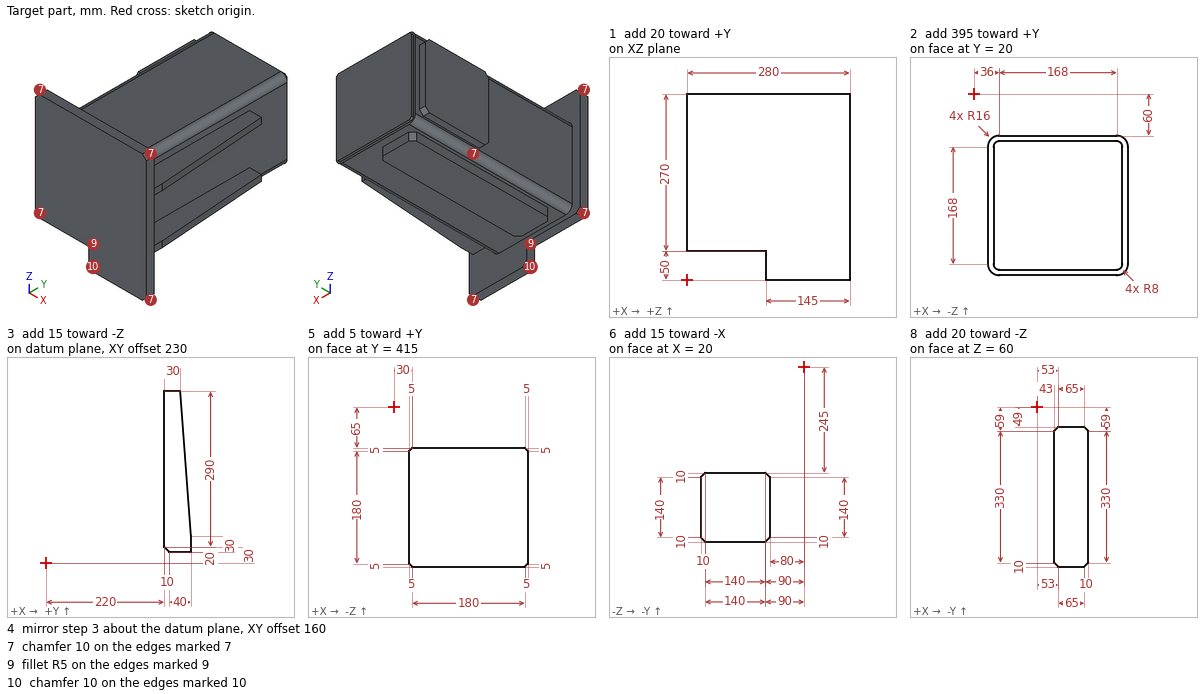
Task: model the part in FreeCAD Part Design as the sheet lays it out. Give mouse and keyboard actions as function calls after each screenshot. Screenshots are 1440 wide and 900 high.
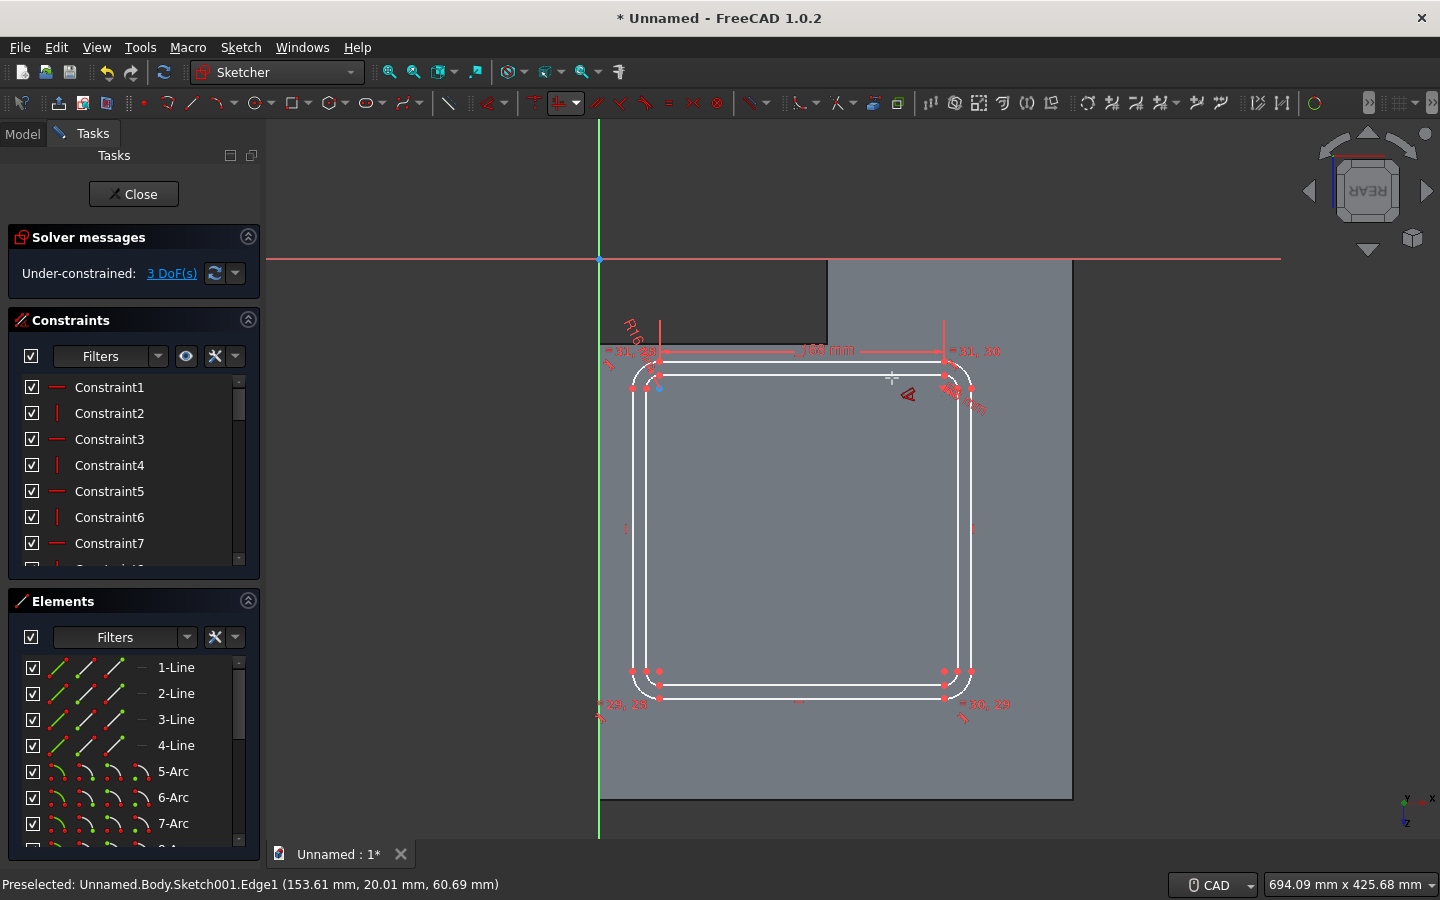
click(633, 474)
click(667, 530)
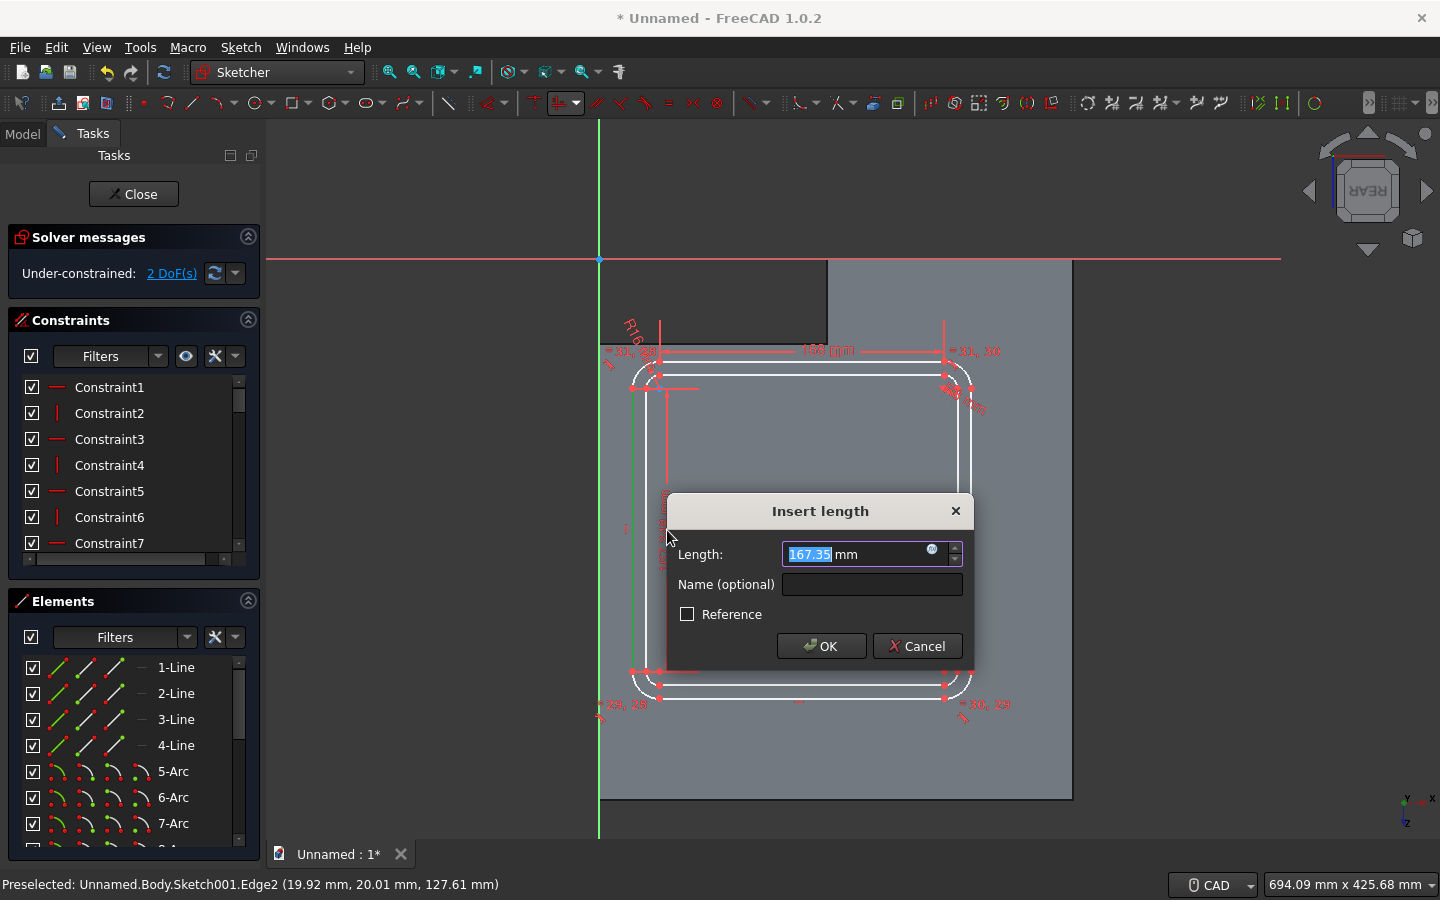
text(168)
key(Return)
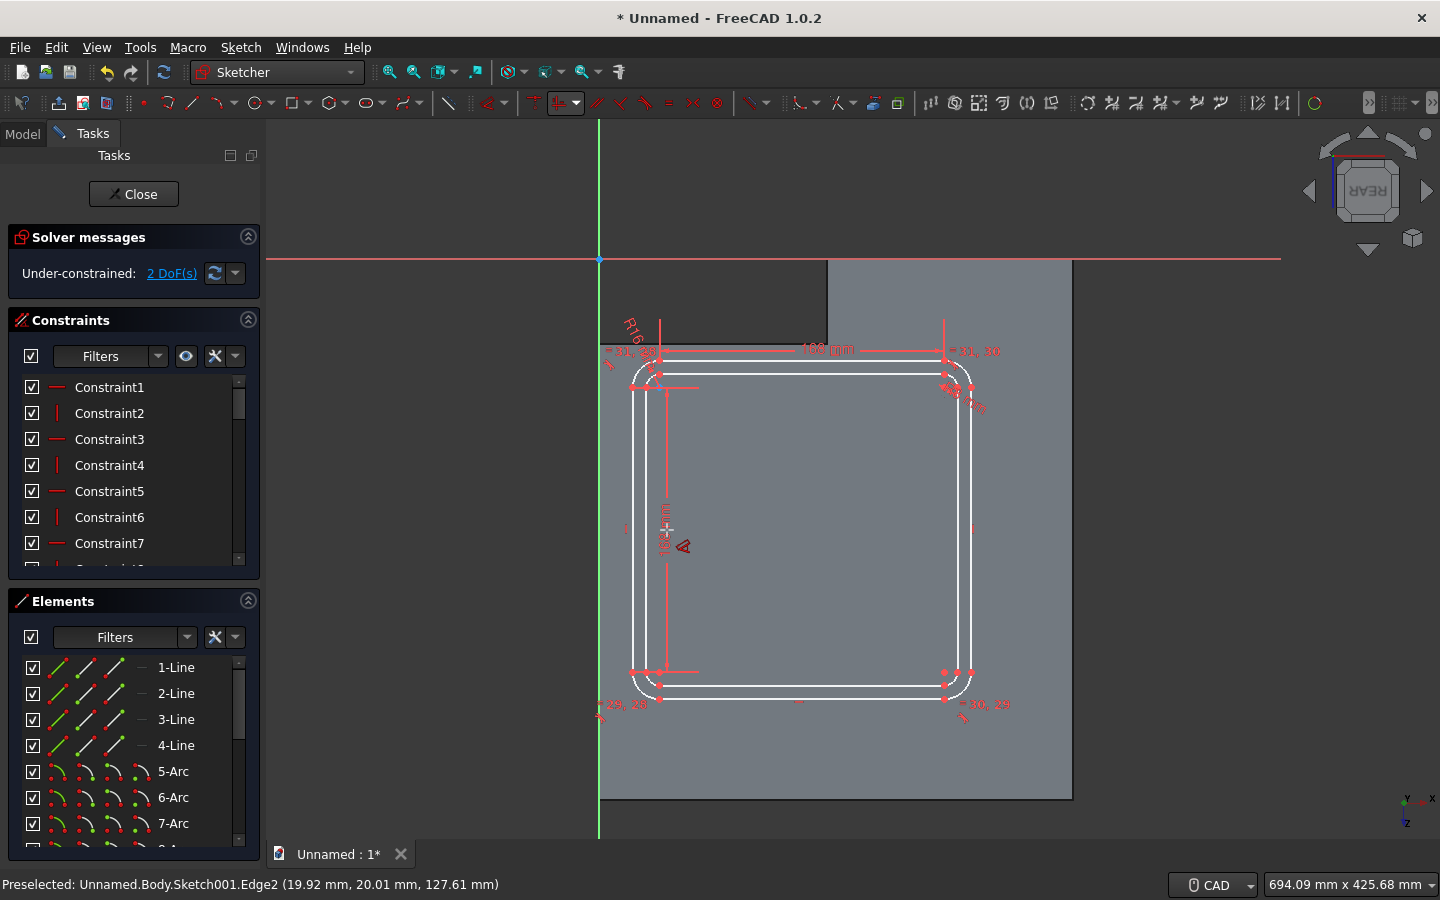
click(944, 361)
click(565, 310)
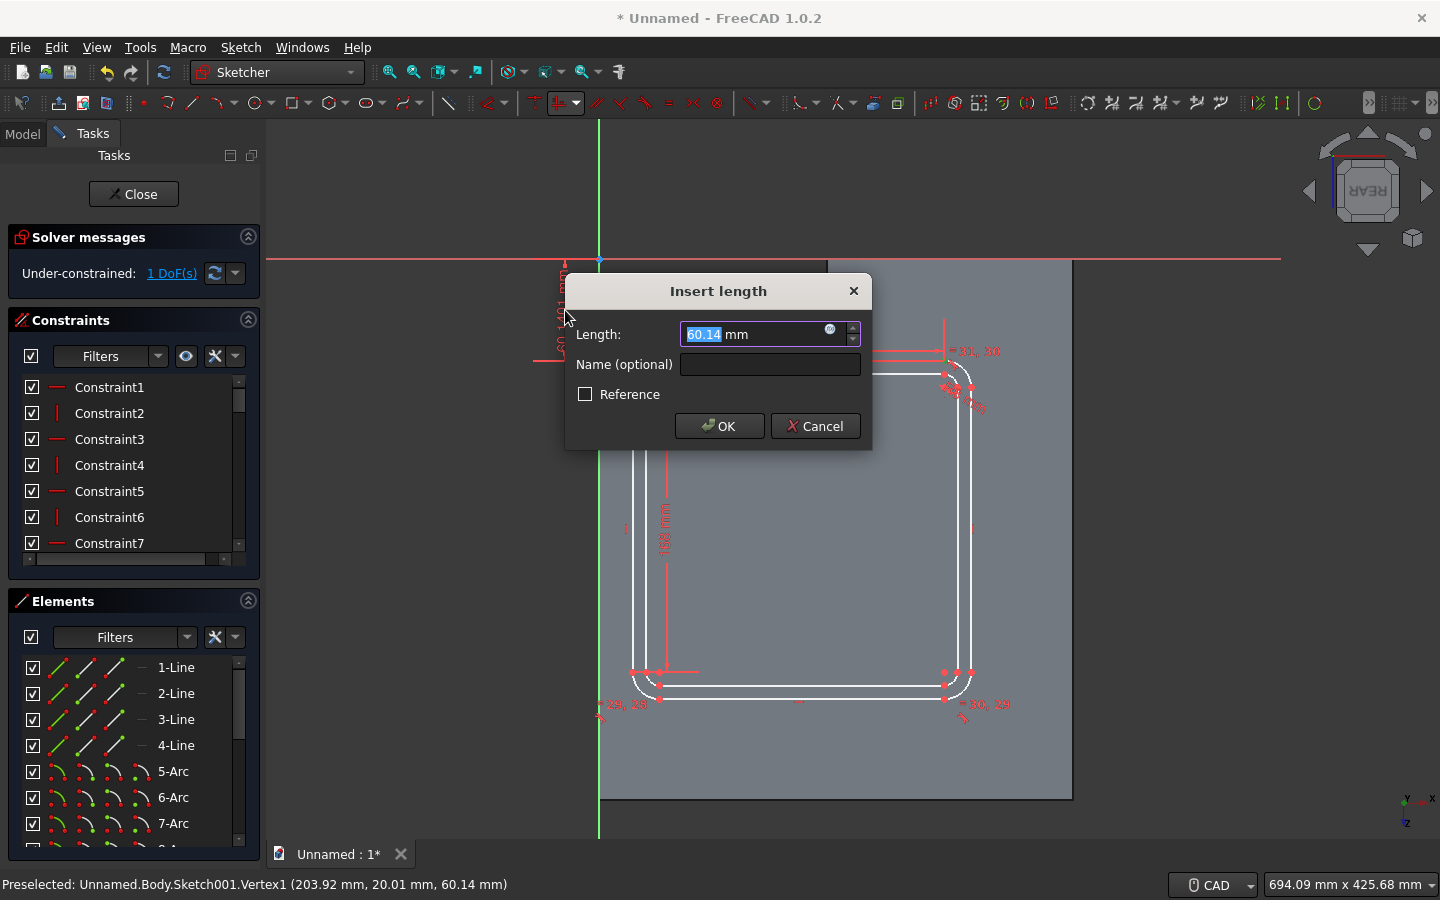
text(60)
key(Return)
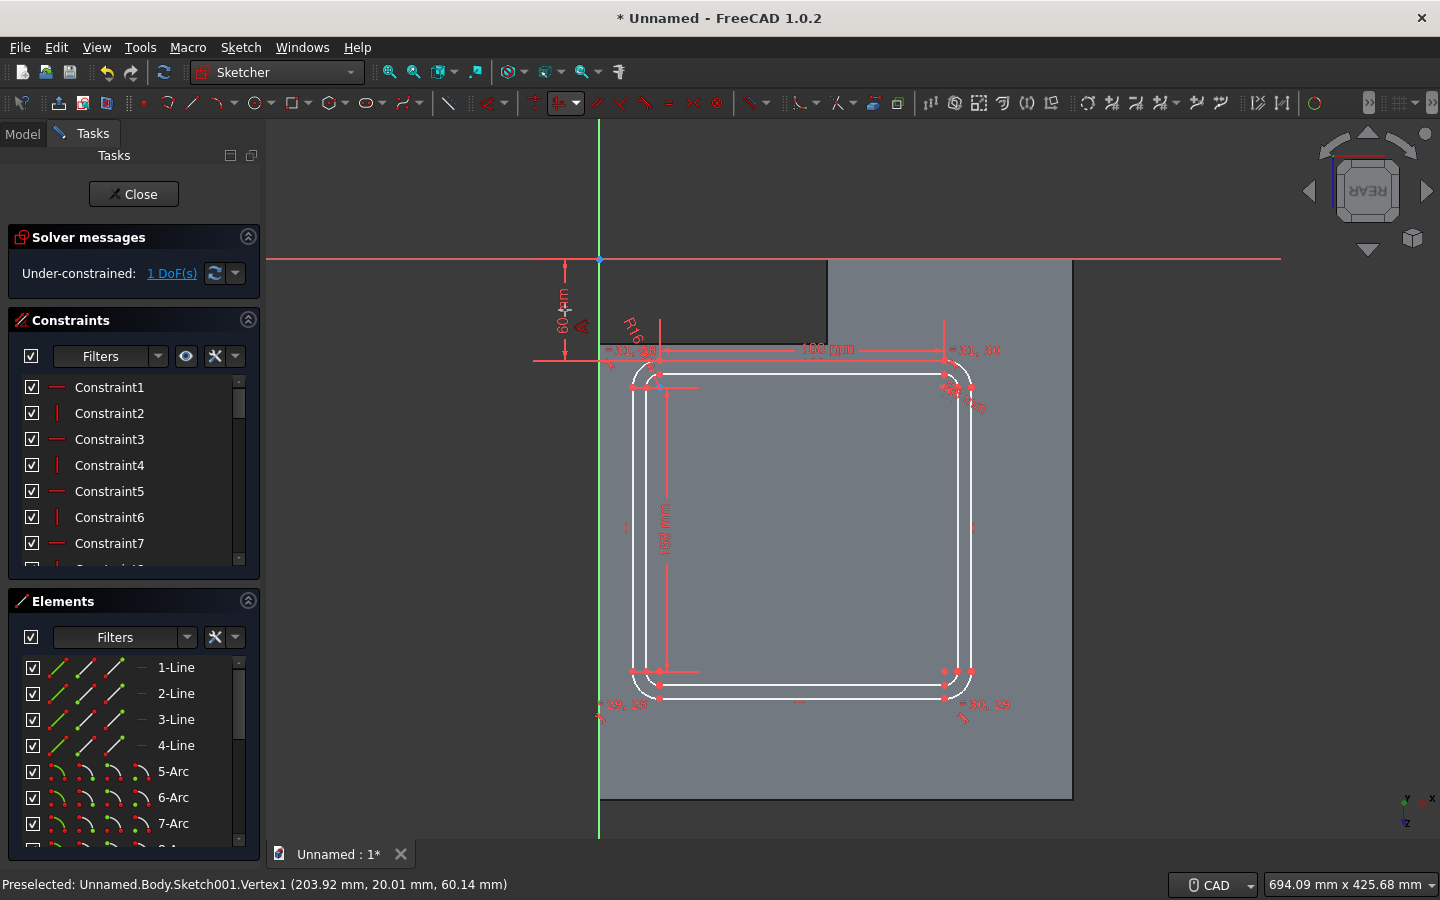
click(660, 361)
click(630, 225)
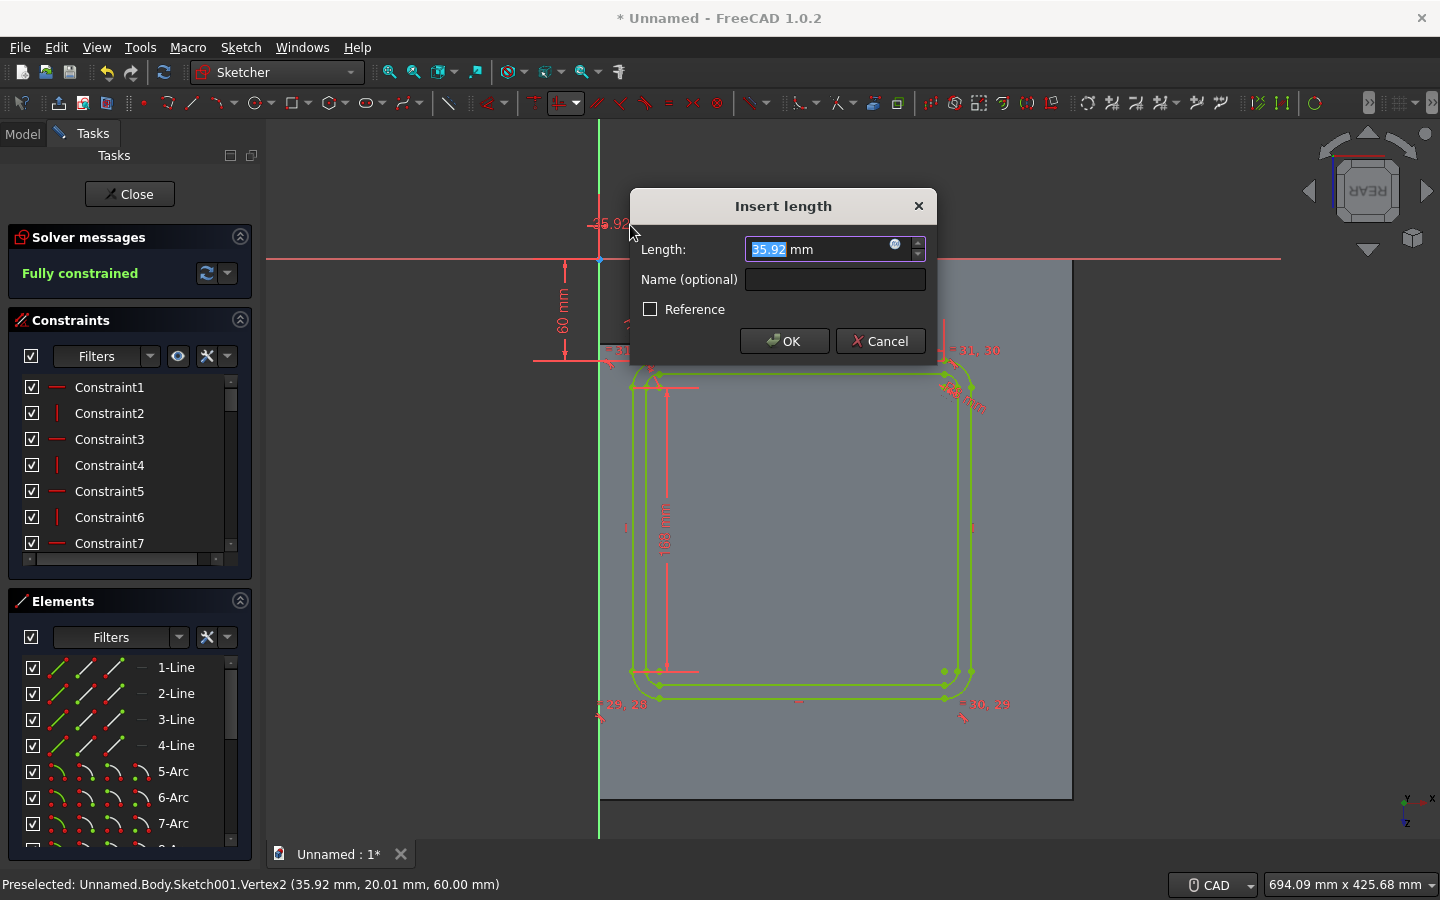
text(36)
key(Return)
key(Escape)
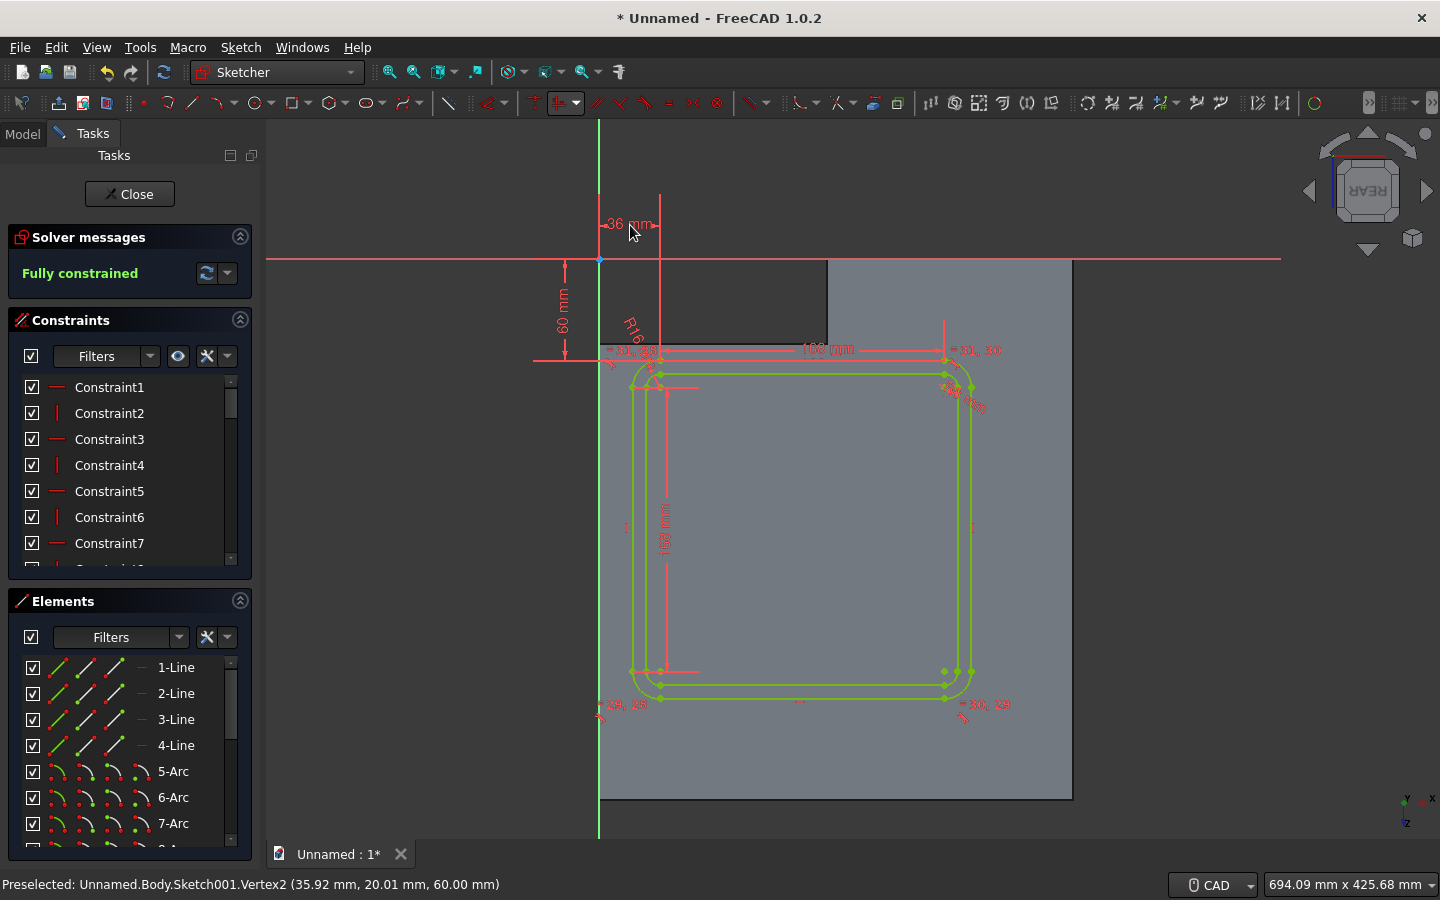
click(130, 194)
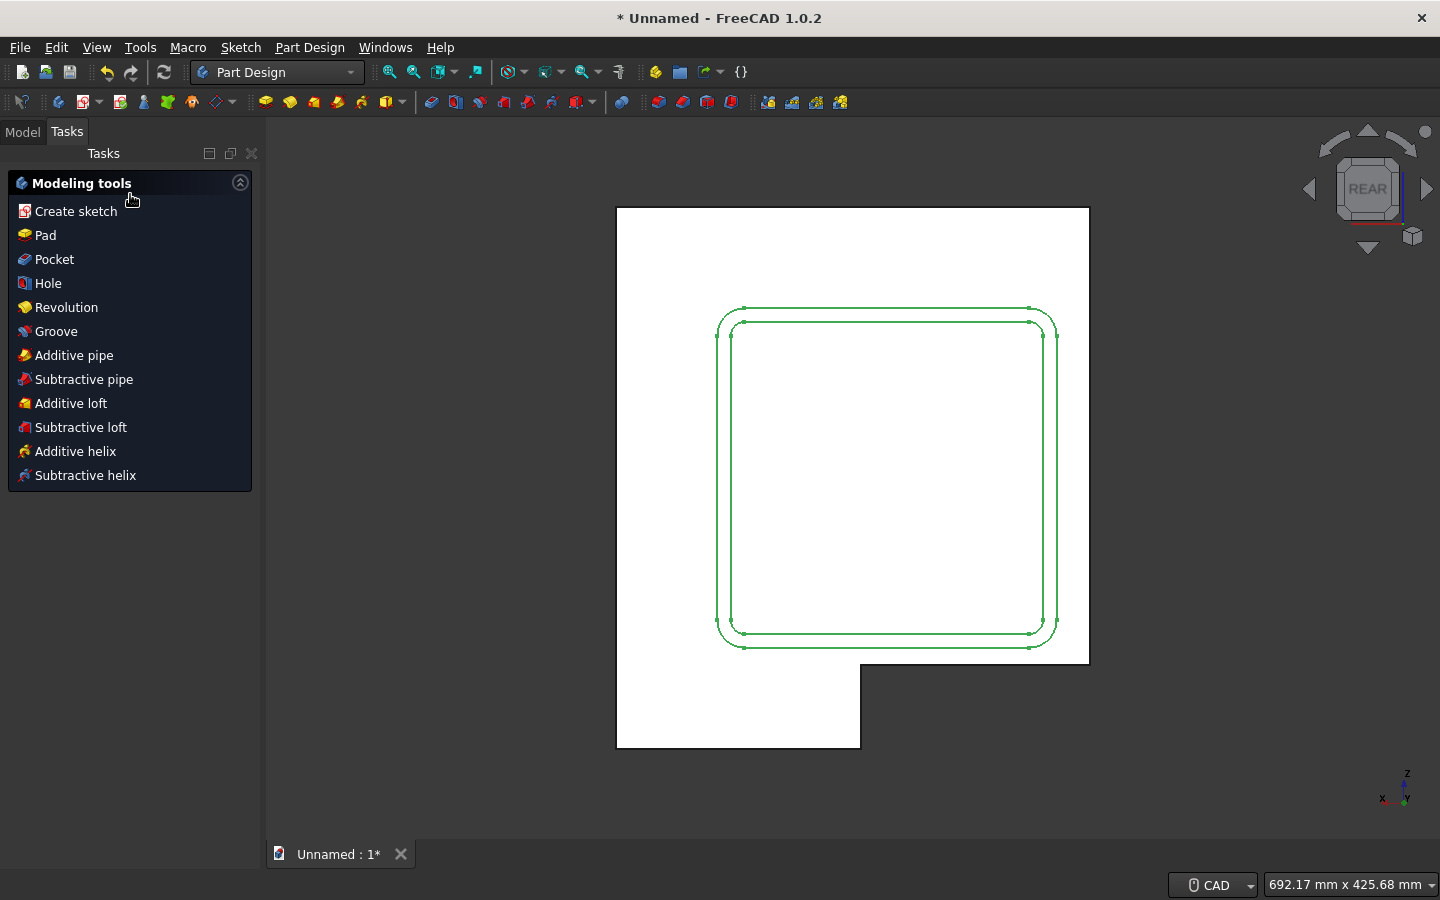
click(266, 102)